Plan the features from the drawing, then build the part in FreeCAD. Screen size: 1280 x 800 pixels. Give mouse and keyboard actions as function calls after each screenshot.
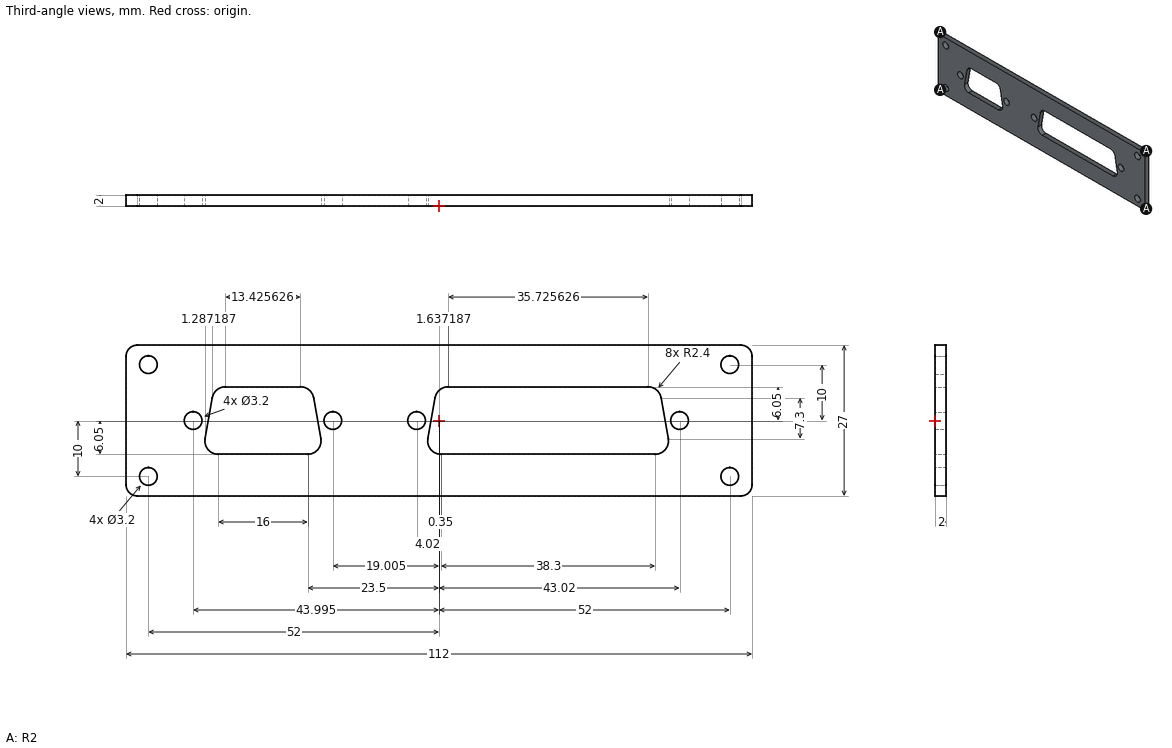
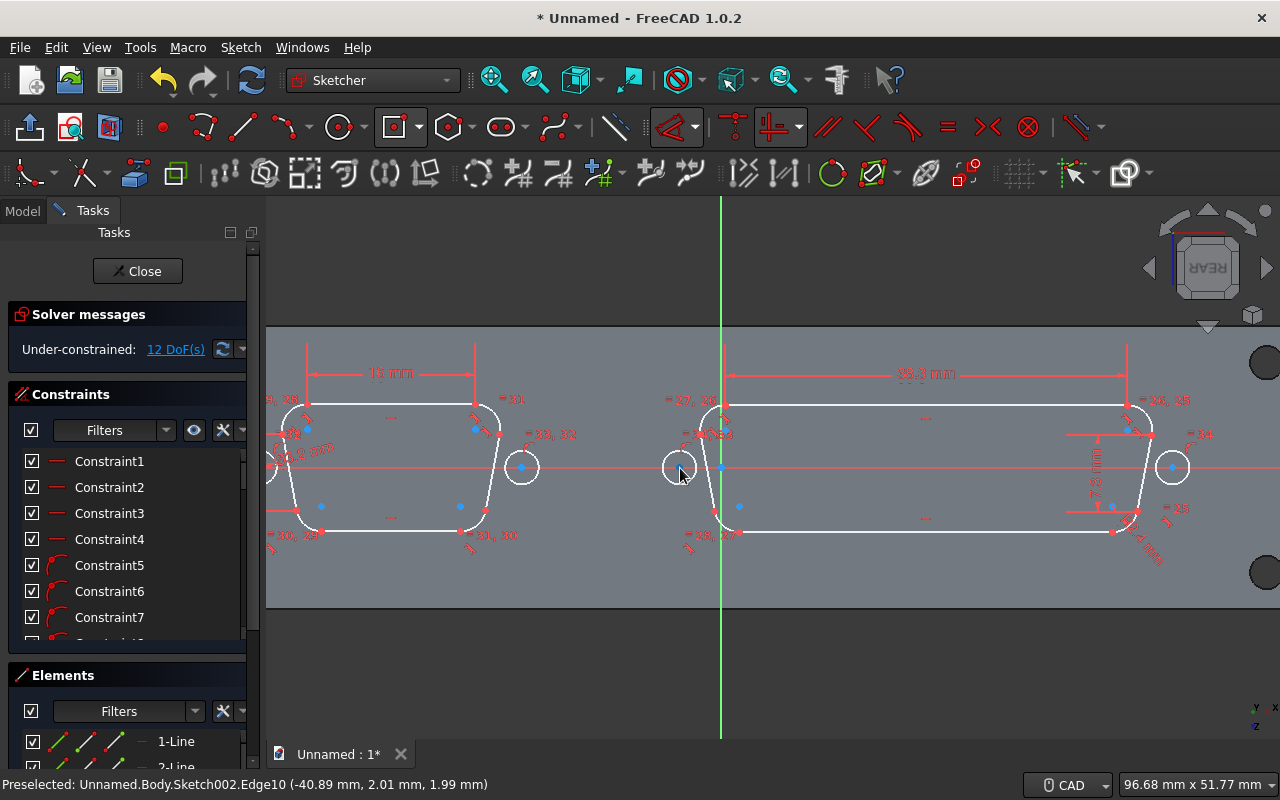
click(680, 468)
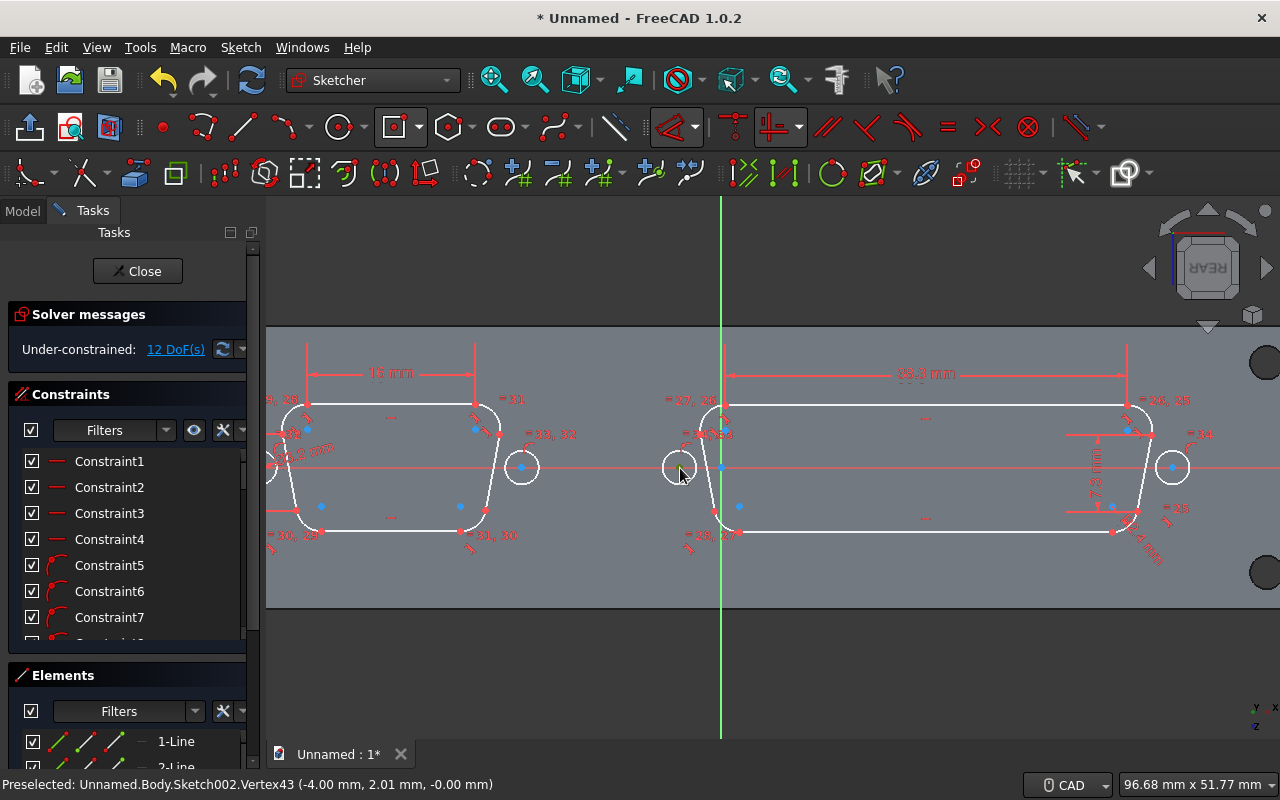
click(698, 128)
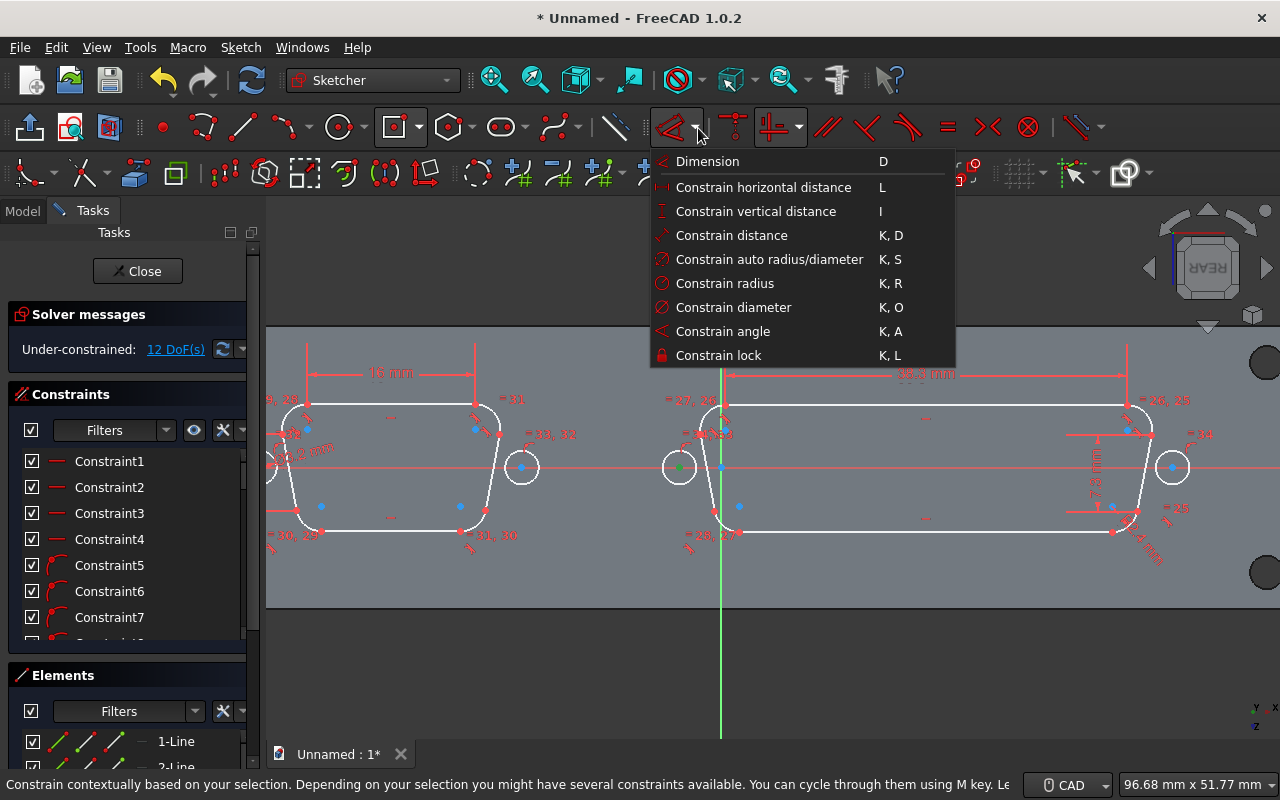
click(803, 187)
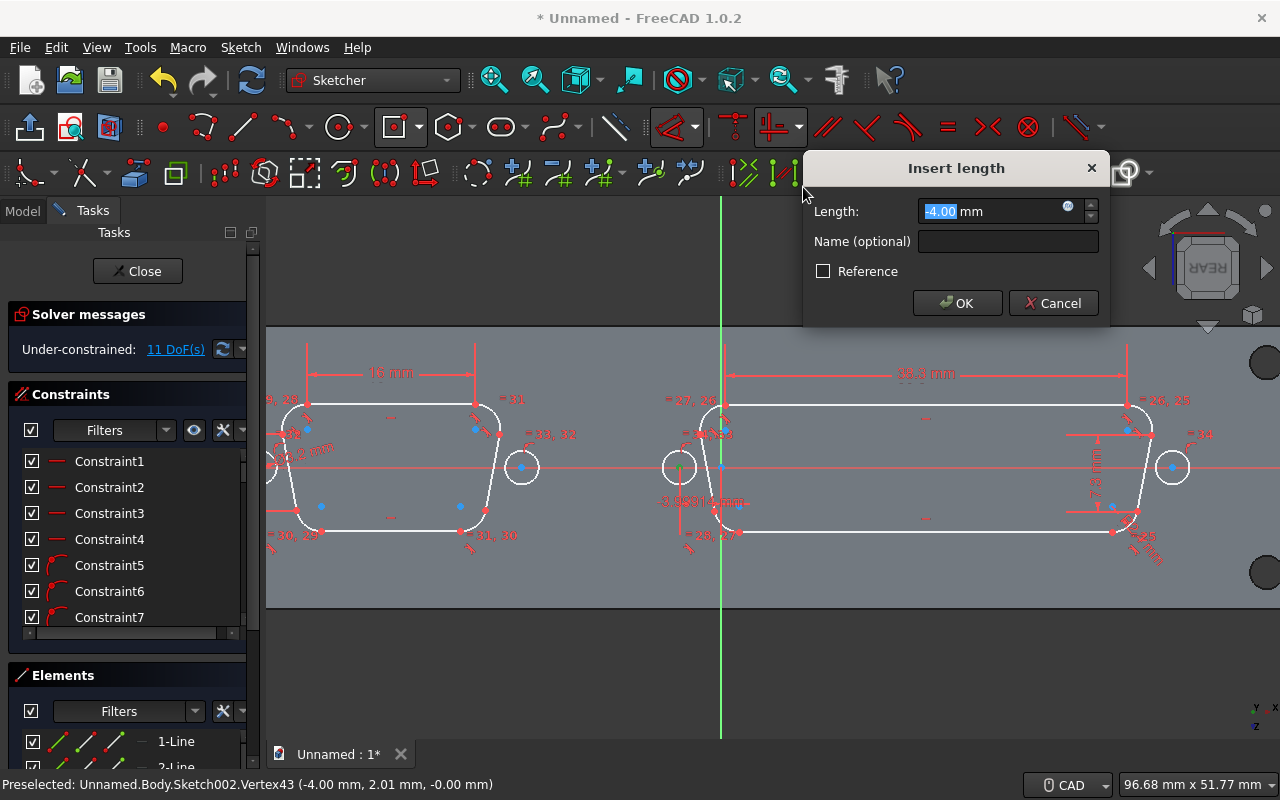
text(-4.02)
key(Return)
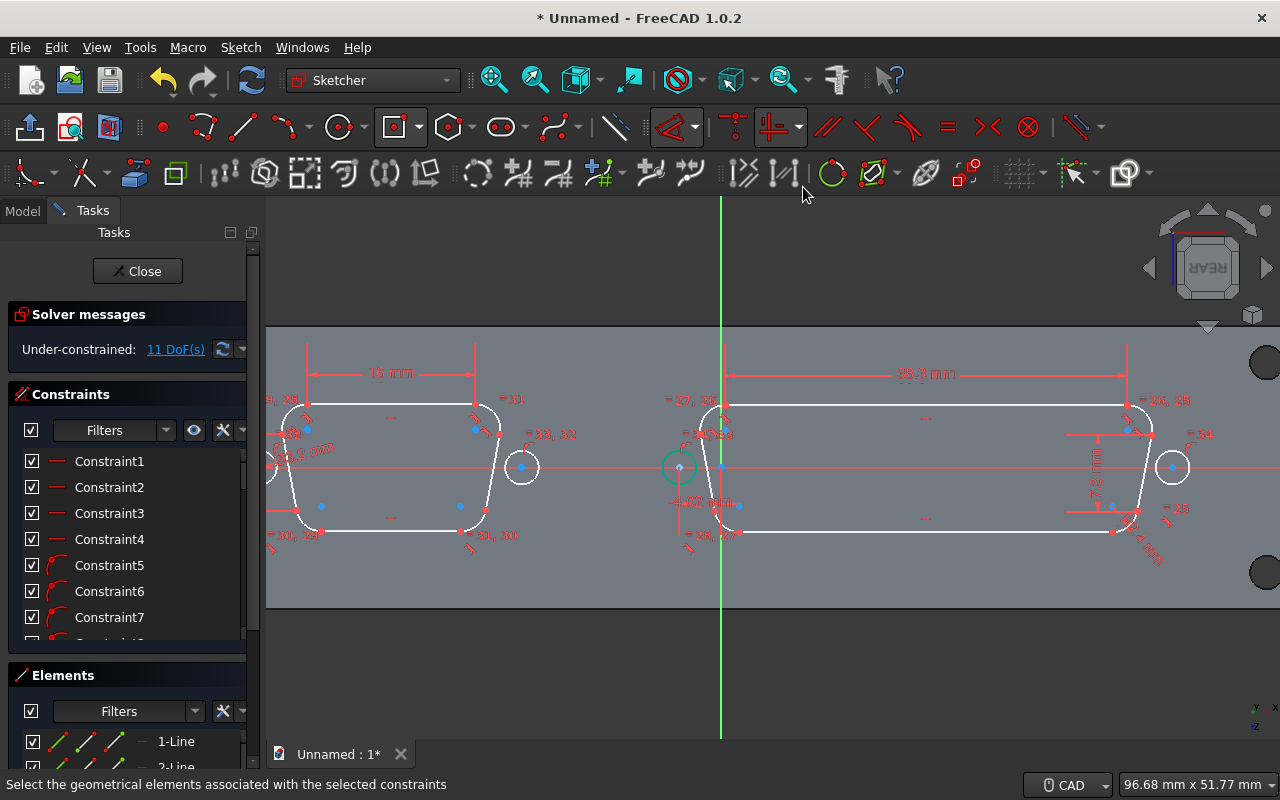
click(740, 532)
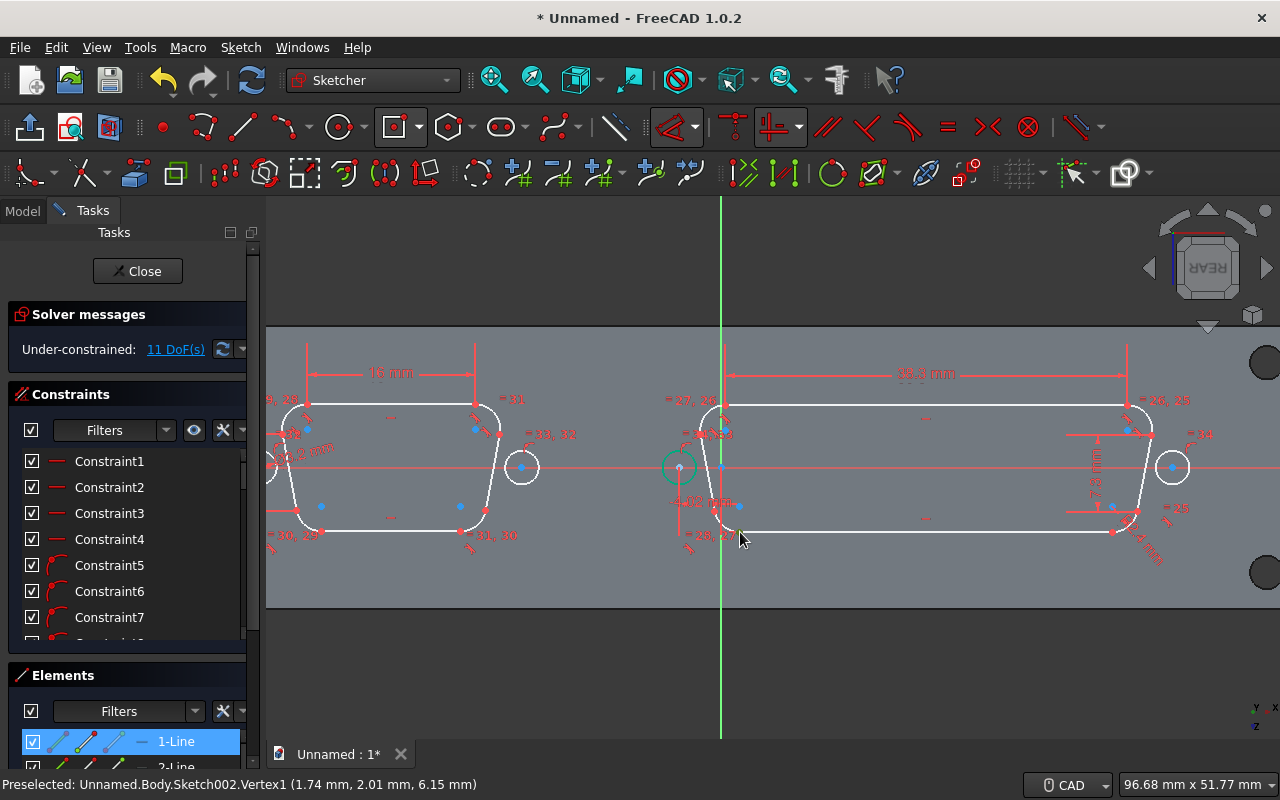
key(i)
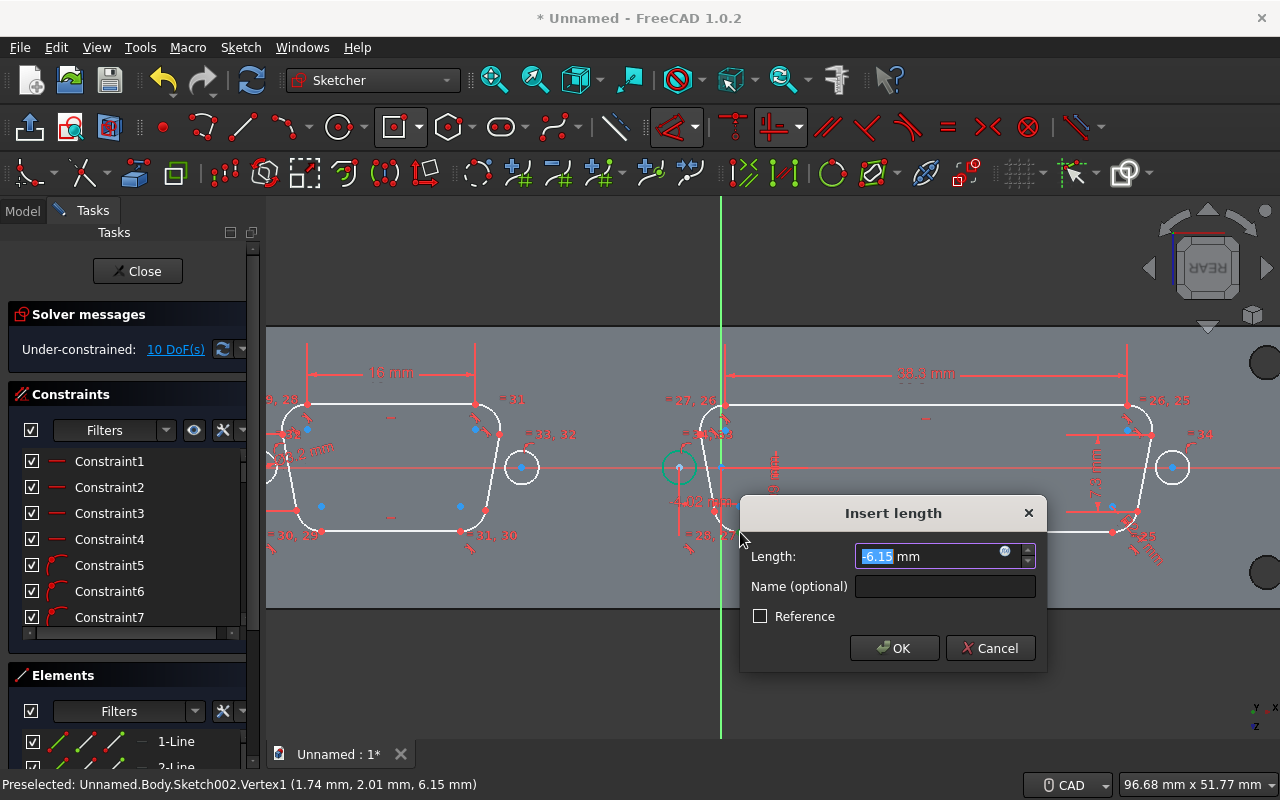
text(-6.05)
key(Return)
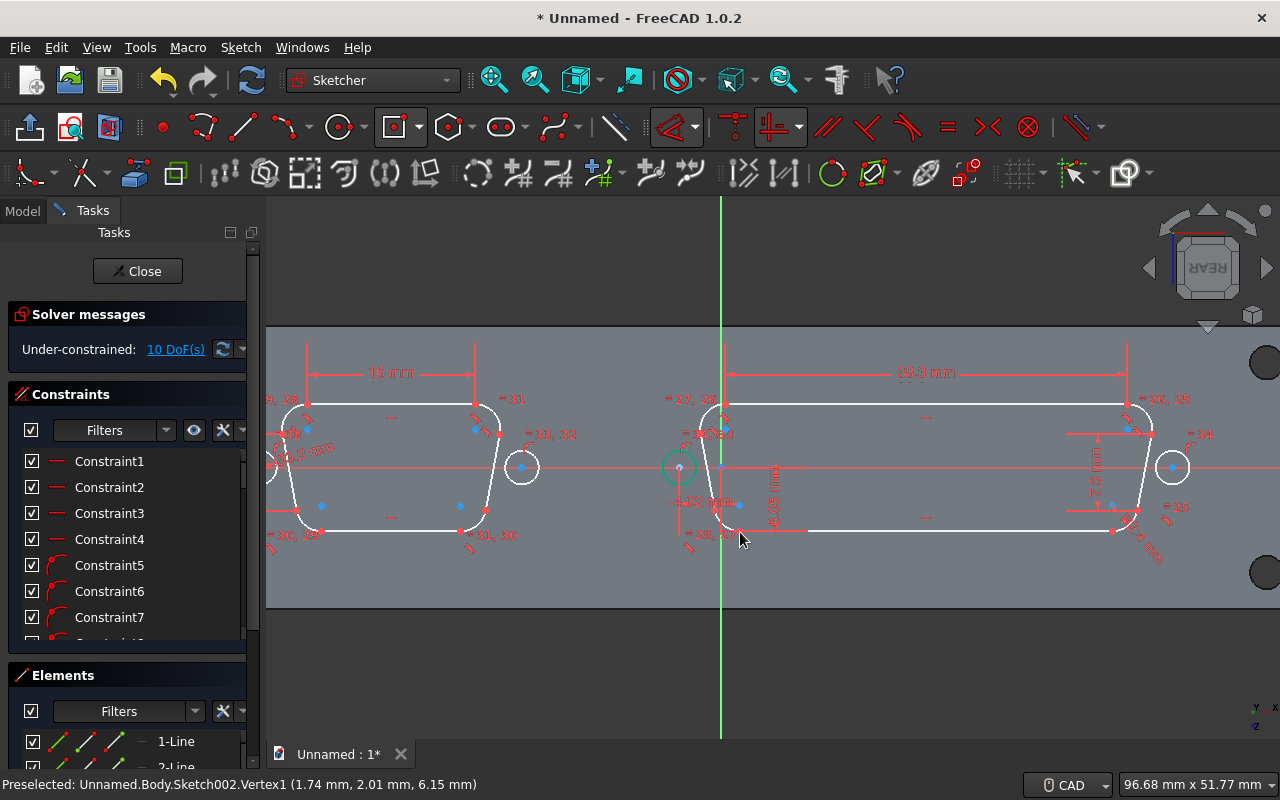
scroll(725, 404, up, 12)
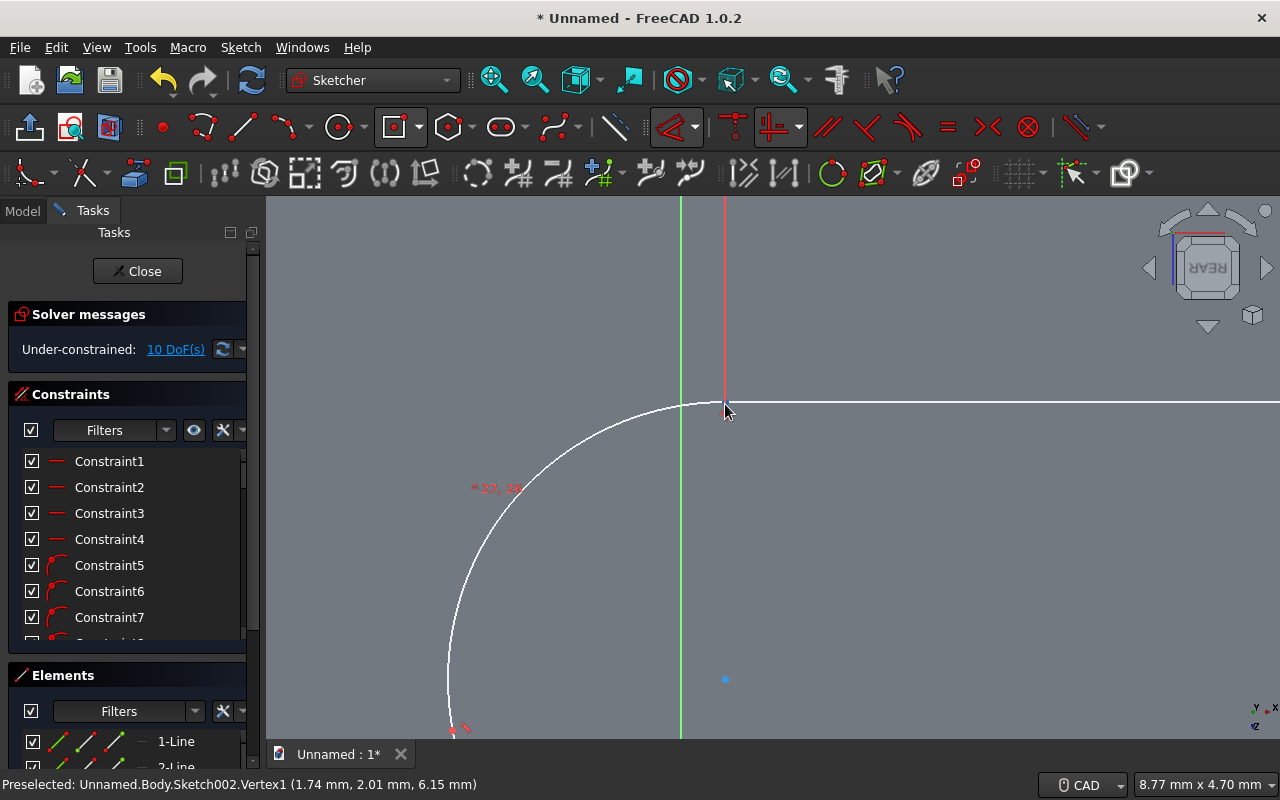
click(725, 402)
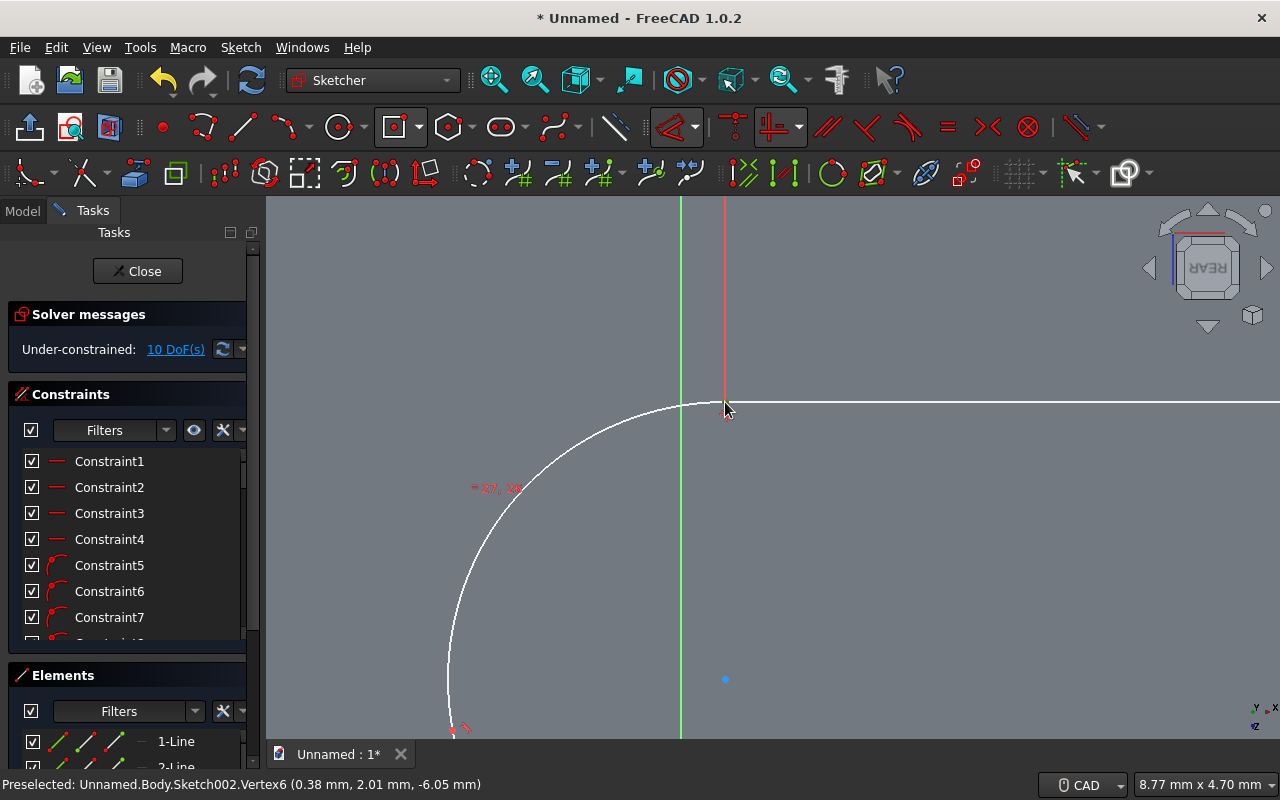
key(l)